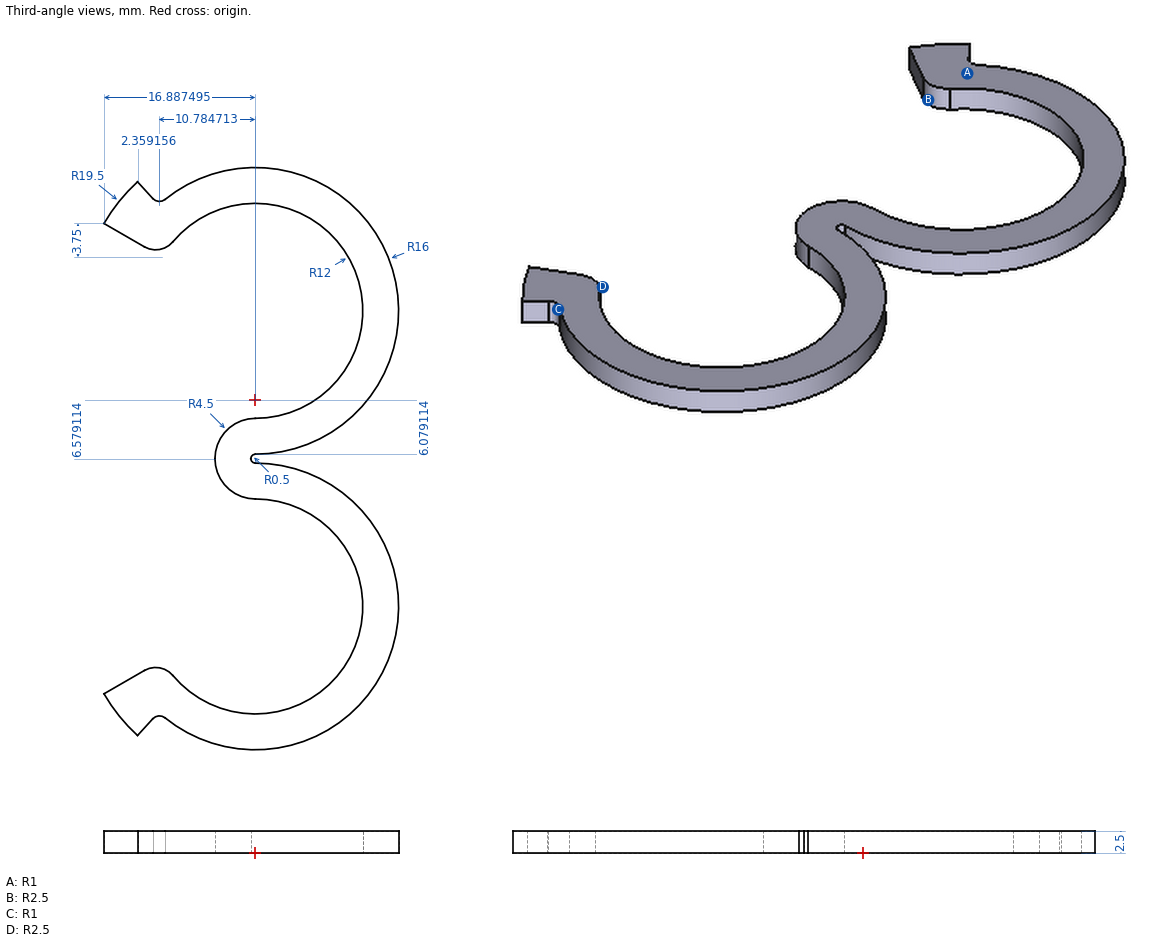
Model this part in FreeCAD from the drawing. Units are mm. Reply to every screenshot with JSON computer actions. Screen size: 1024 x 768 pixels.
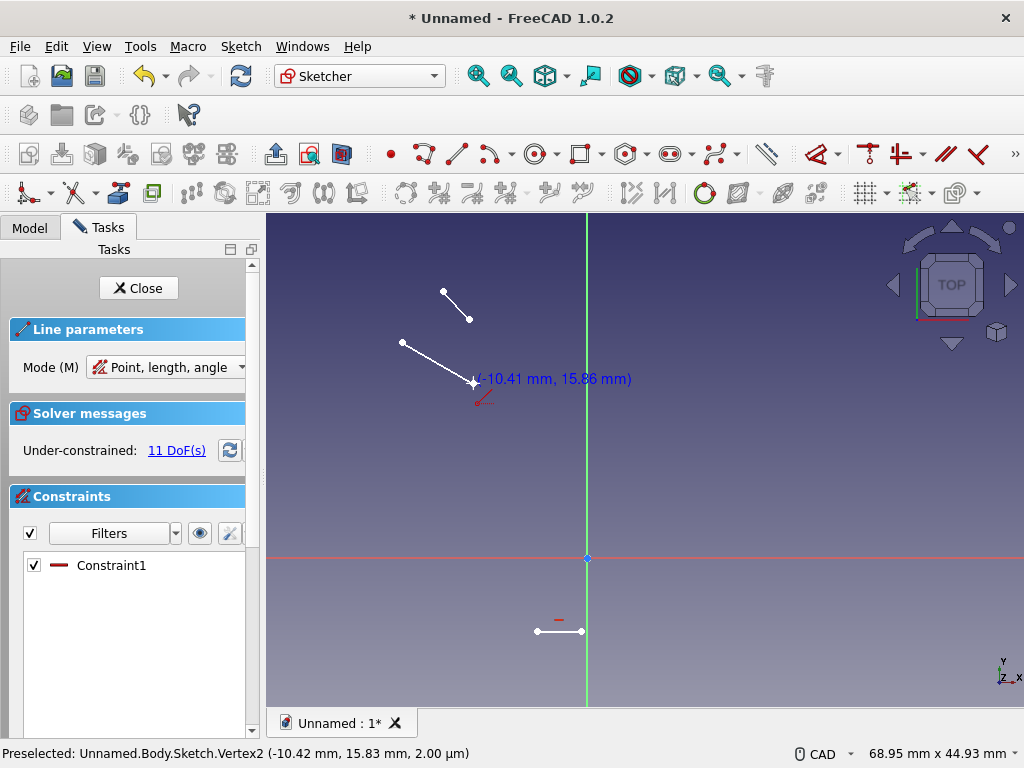
{"action": "key", "text": "g 3 a"}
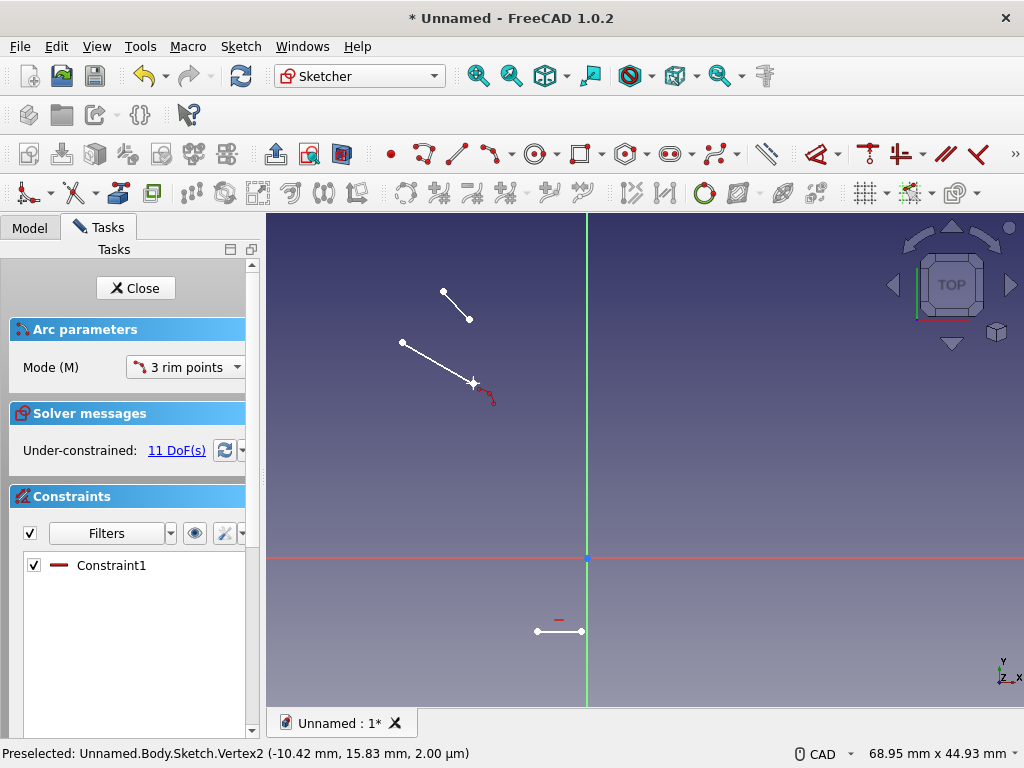
{"action": "scroll", "coordinate": [582, 631], "scroll_direction": "up", "scroll_amount": 6}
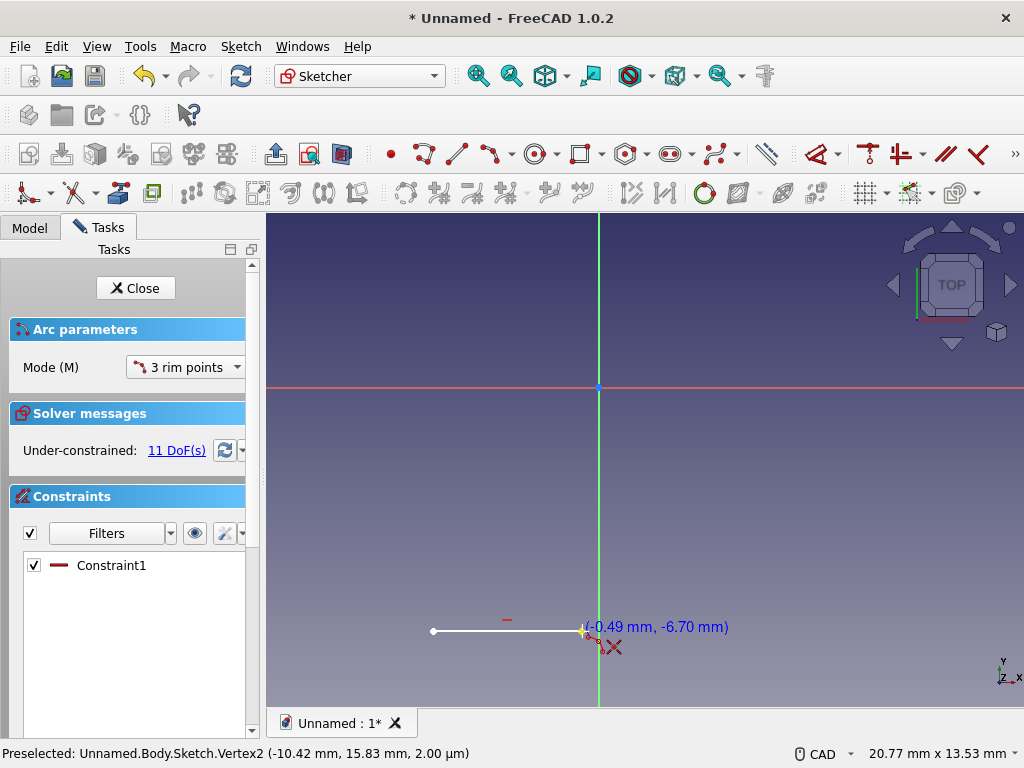
{"action": "left_click", "coordinate": [581, 631]}
{"action": "left_click", "coordinate": [599, 610]}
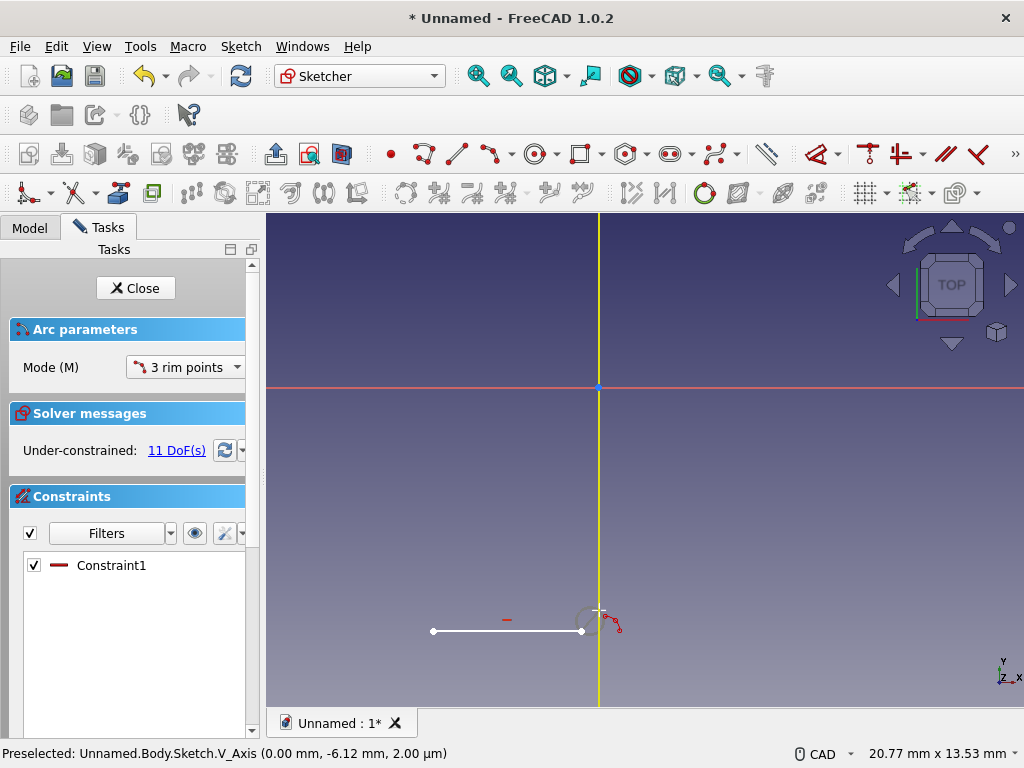
{"action": "scroll", "coordinate": [586, 615], "scroll_direction": "up", "scroll_amount": 6}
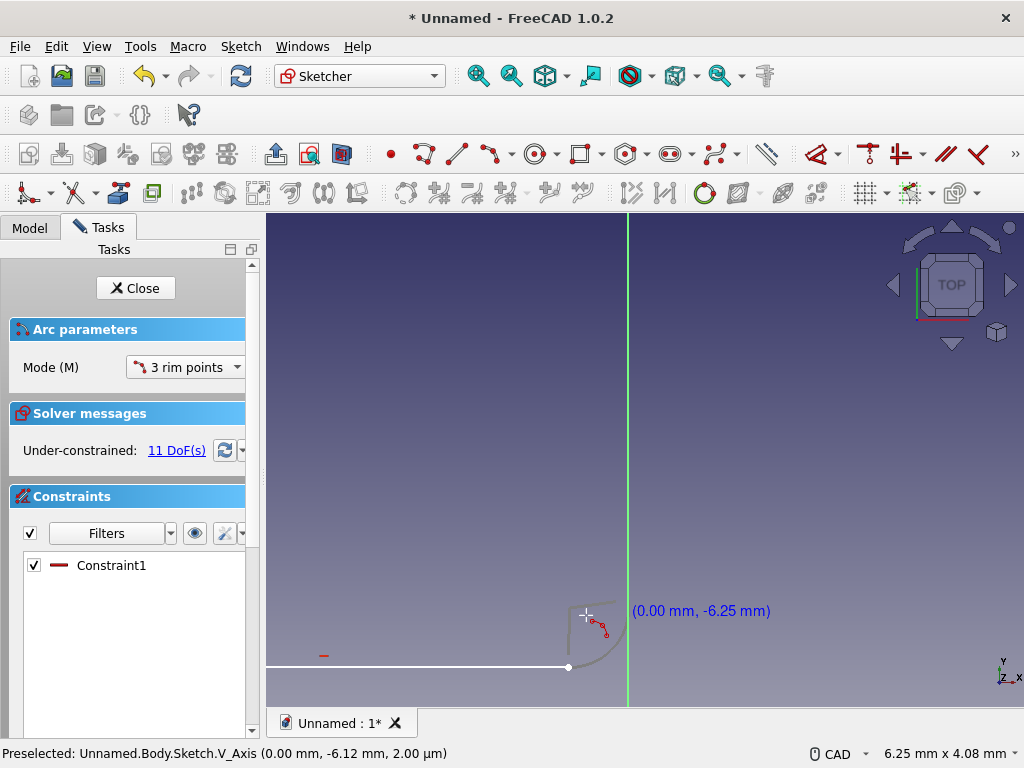
{"action": "left_click", "coordinate": [585, 613]}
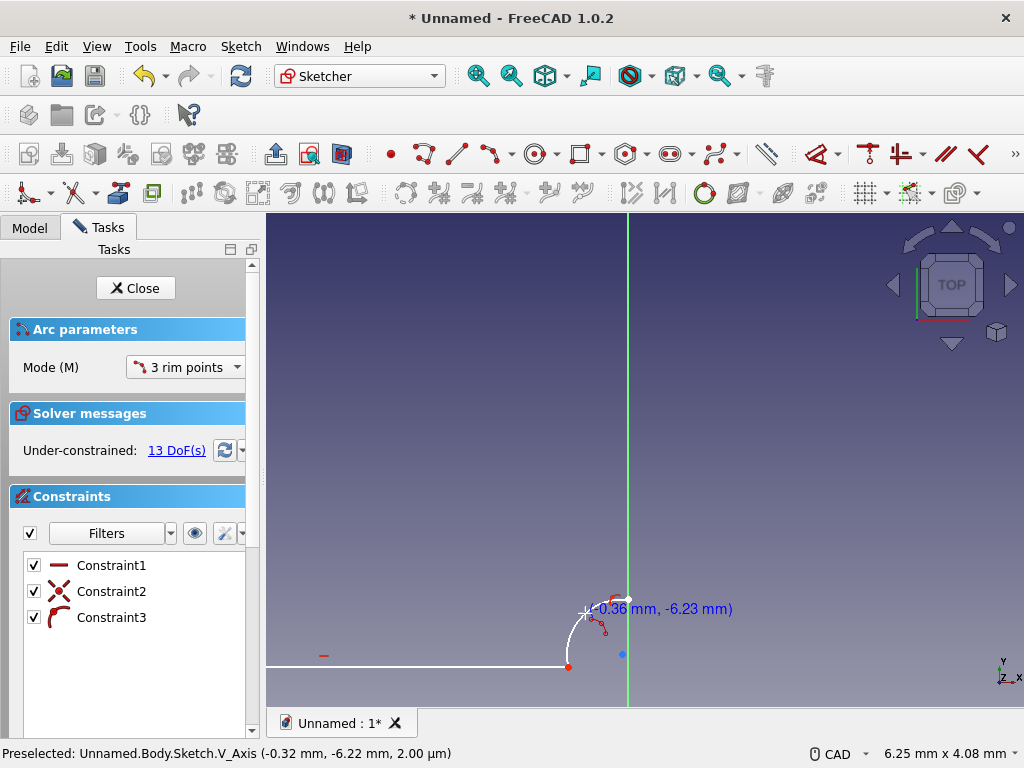
{"action": "scroll", "coordinate": [583, 627], "scroll_direction": "down", "scroll_amount": 12}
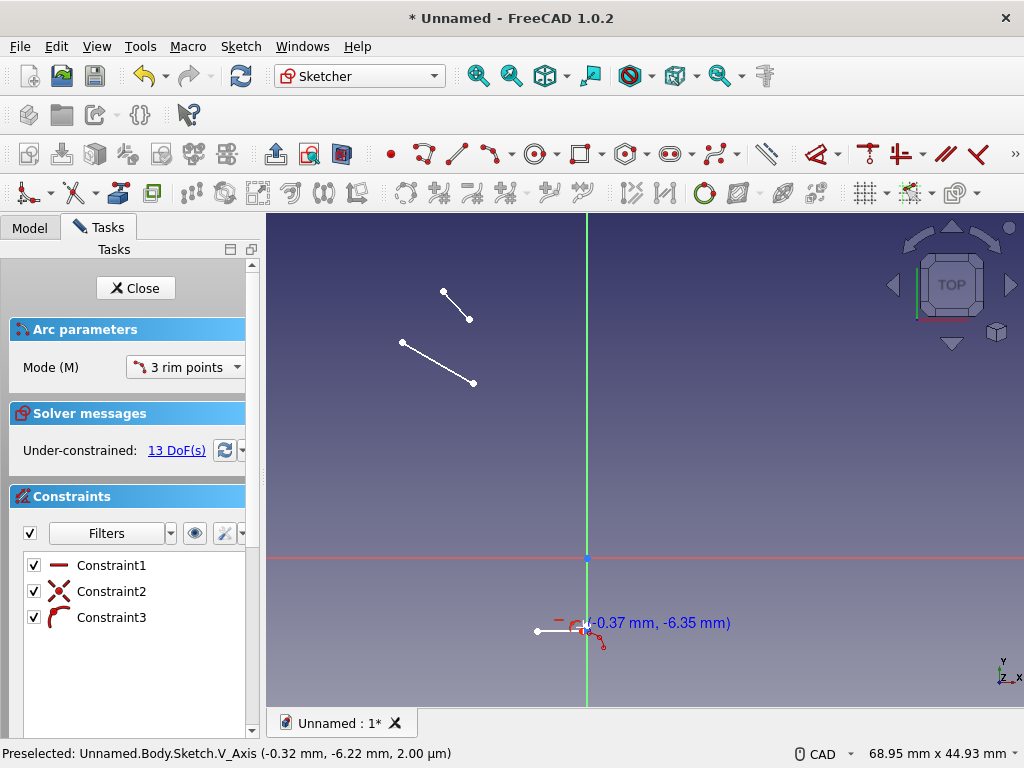
{"action": "scroll", "coordinate": [587, 625], "scroll_direction": "up", "scroll_amount": 6}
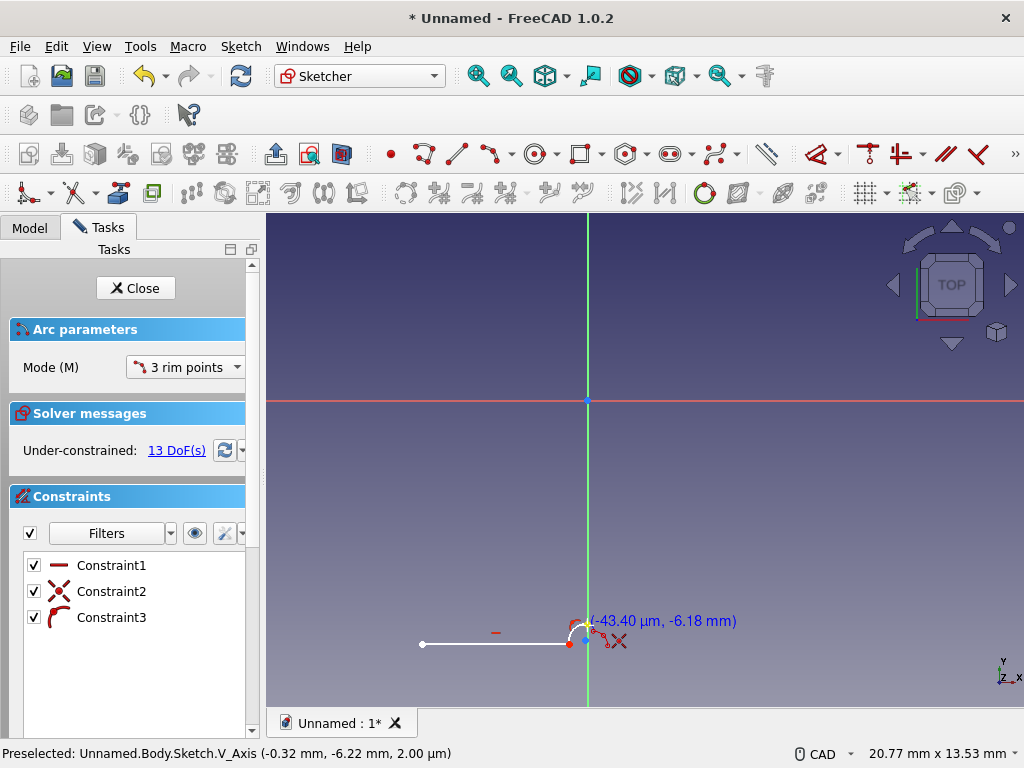
{"action": "left_click", "coordinate": [588, 624]}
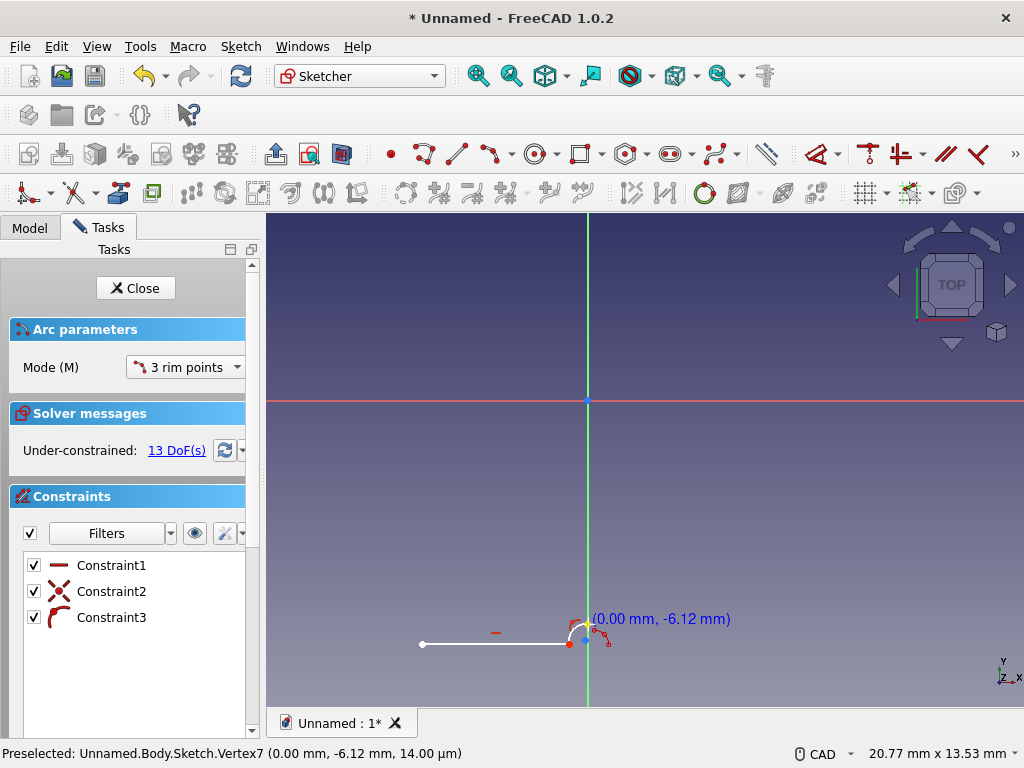
{"action": "scroll", "coordinate": [587, 625], "scroll_direction": "down", "scroll_amount": 6}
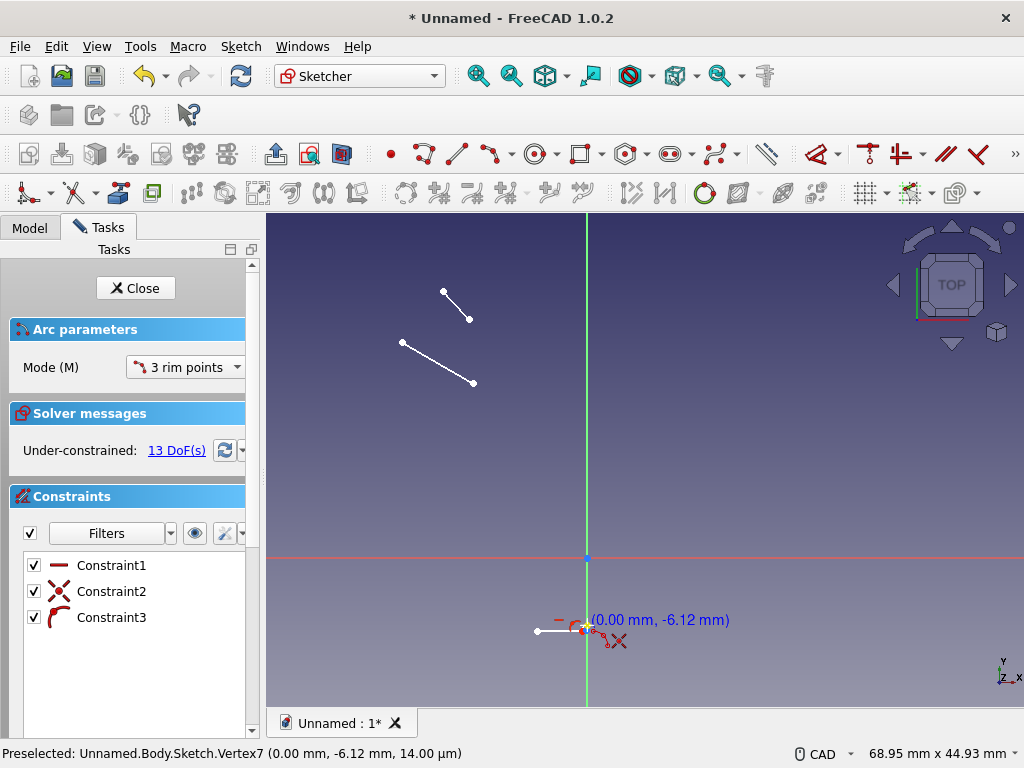
{"action": "left_click", "coordinate": [469, 320]}
{"action": "left_click", "coordinate": [751, 385]}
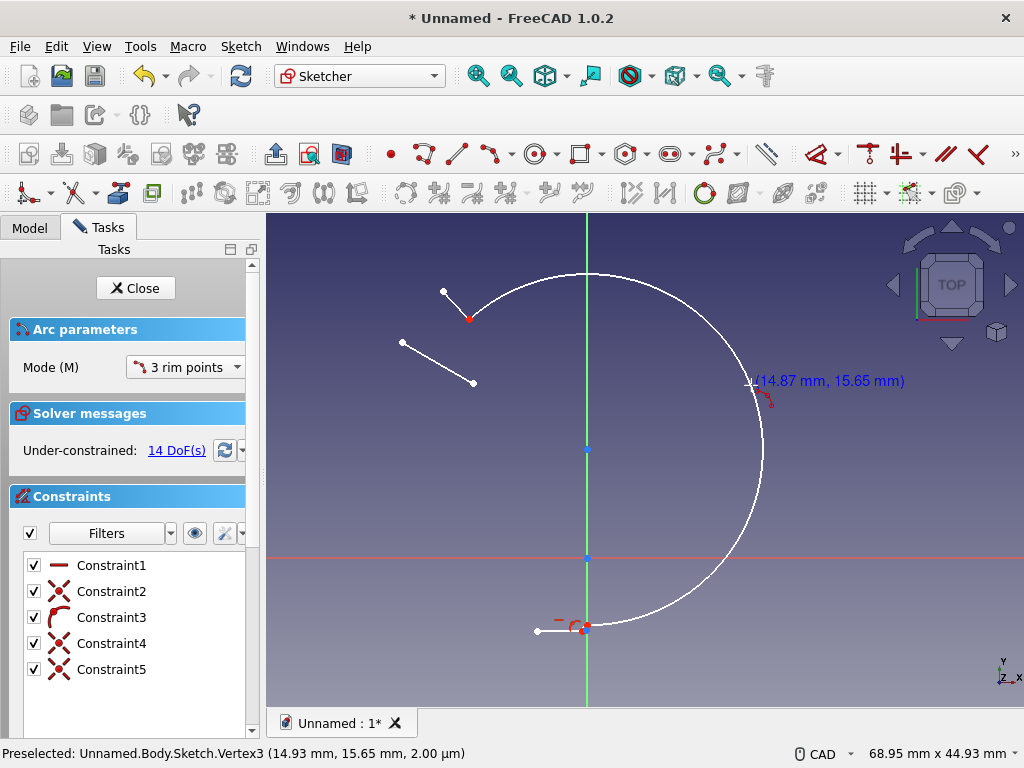
{"action": "left_click", "coordinate": [443, 292]}
{"action": "left_click", "coordinate": [402, 343]}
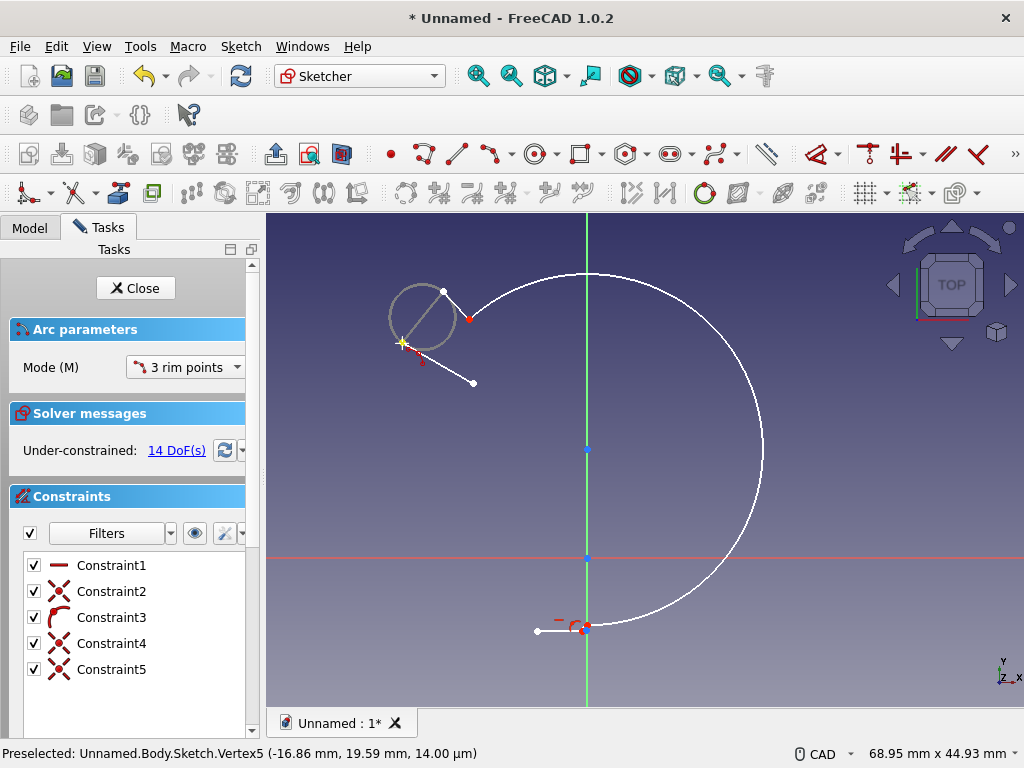
{"action": "scroll", "coordinate": [420, 315], "scroll_direction": "up", "scroll_amount": 10}